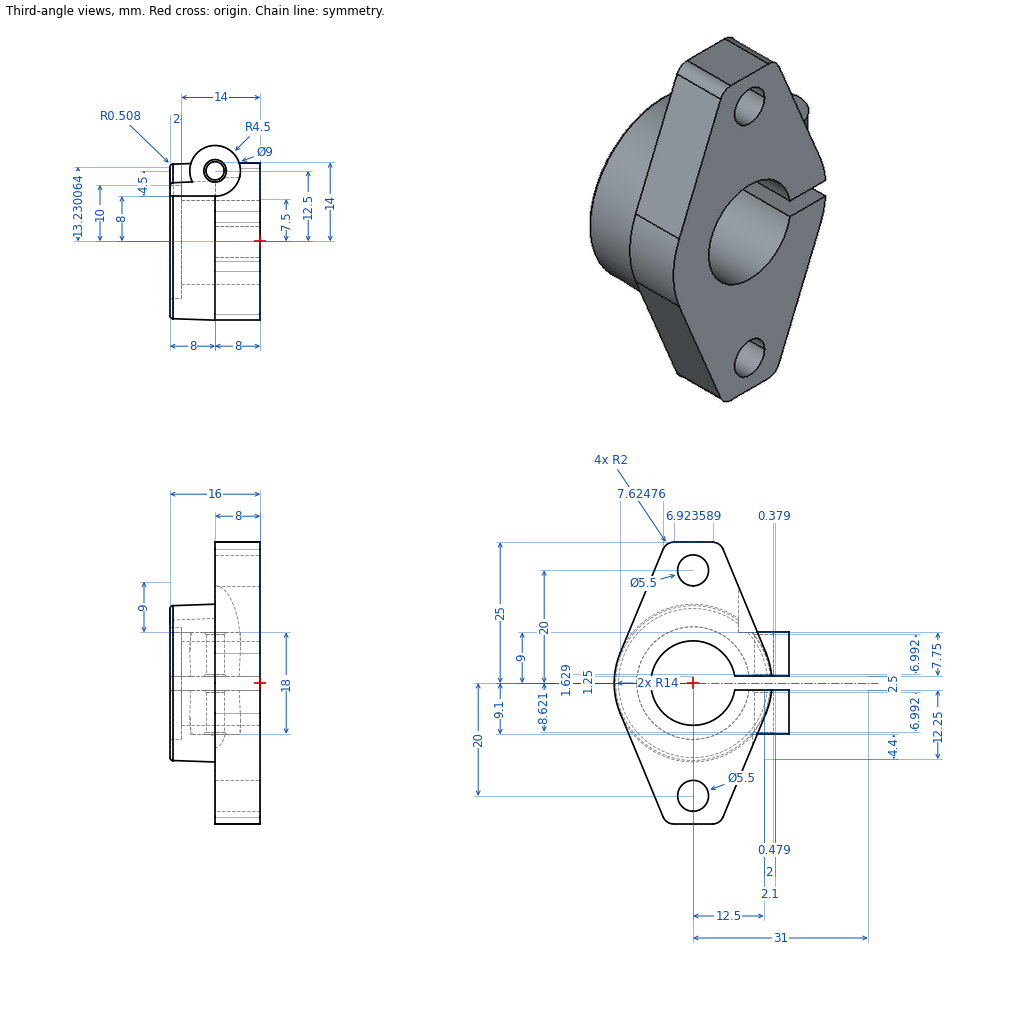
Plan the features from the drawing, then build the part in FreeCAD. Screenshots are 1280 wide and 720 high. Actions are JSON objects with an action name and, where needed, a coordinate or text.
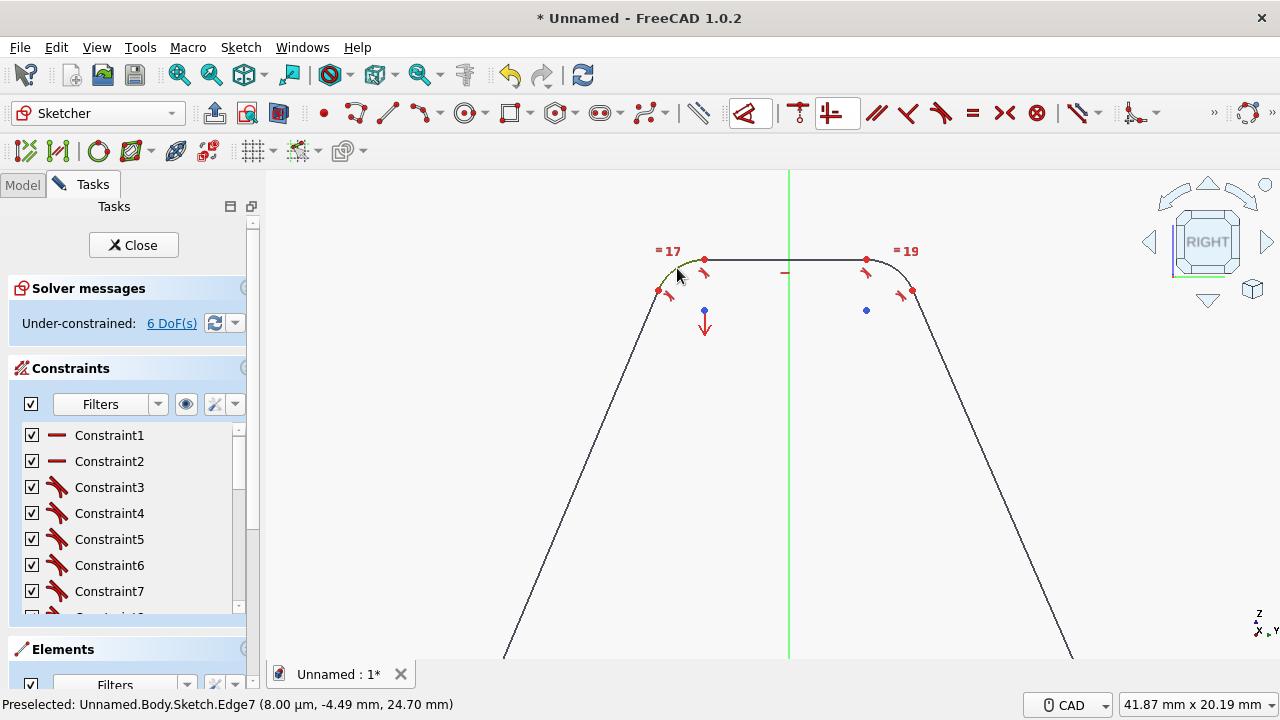
{"action": "key", "text": "k r"}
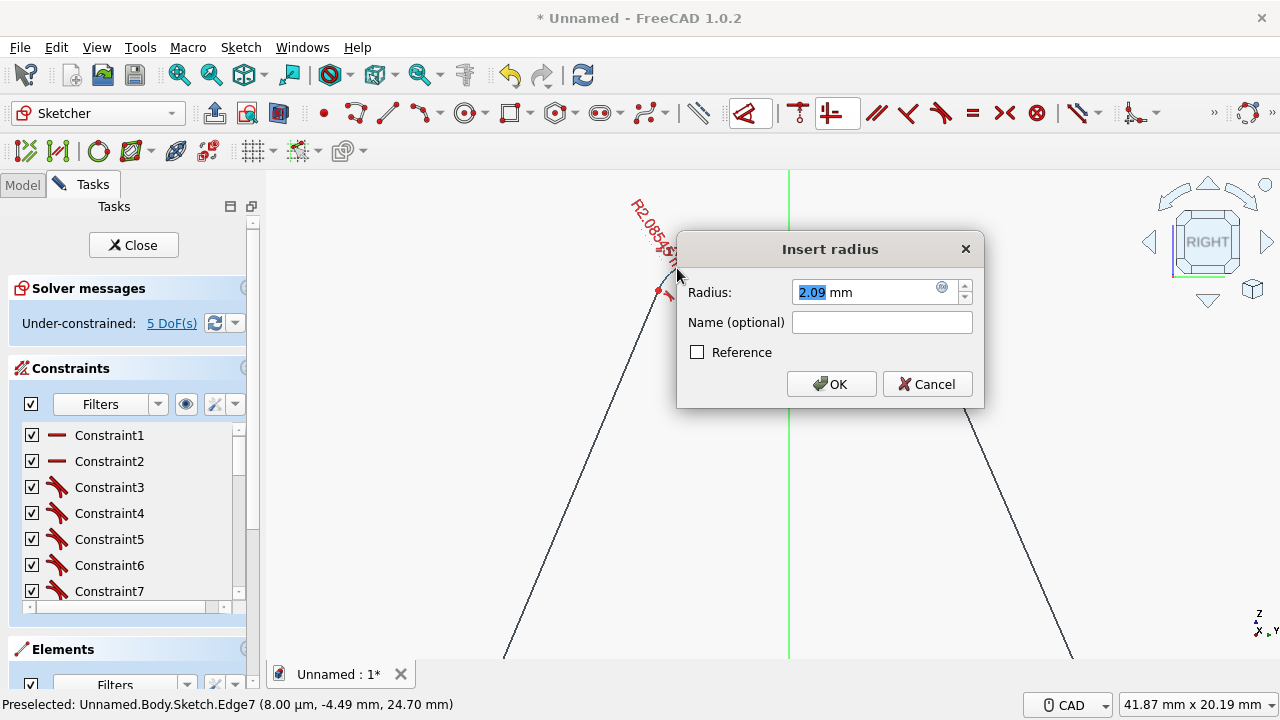
{"action": "type", "text": "2"}
{"action": "key", "text": "Return"}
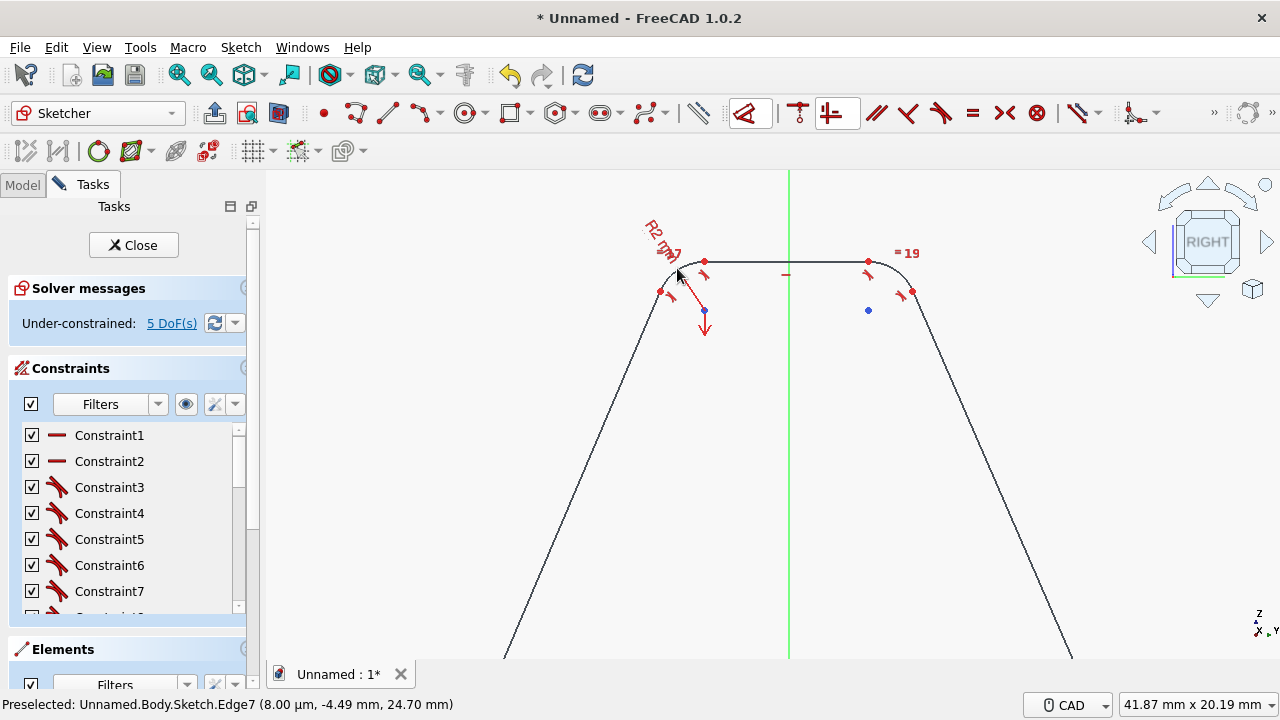
{"action": "scroll", "coordinate": [677, 267], "scroll_direction": "down", "scroll_amount": 7}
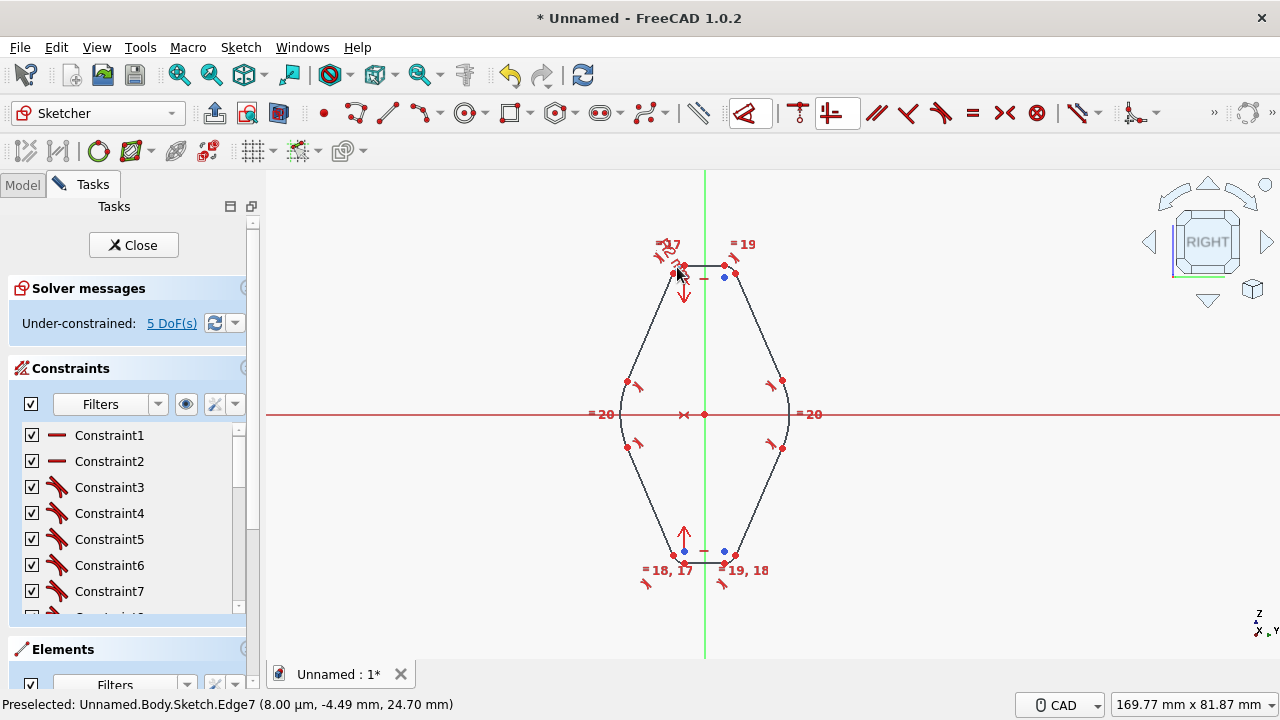
{"action": "left_click", "coordinate": [621, 401]}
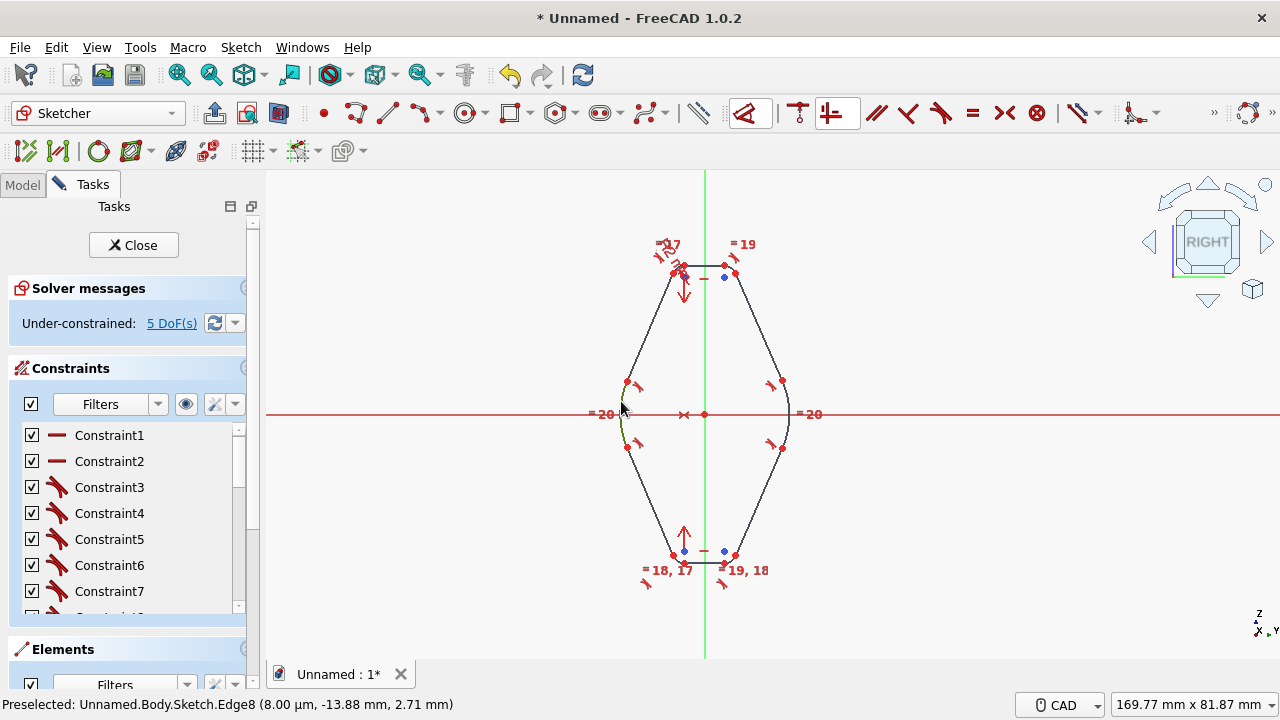
{"action": "key", "text": "k r"}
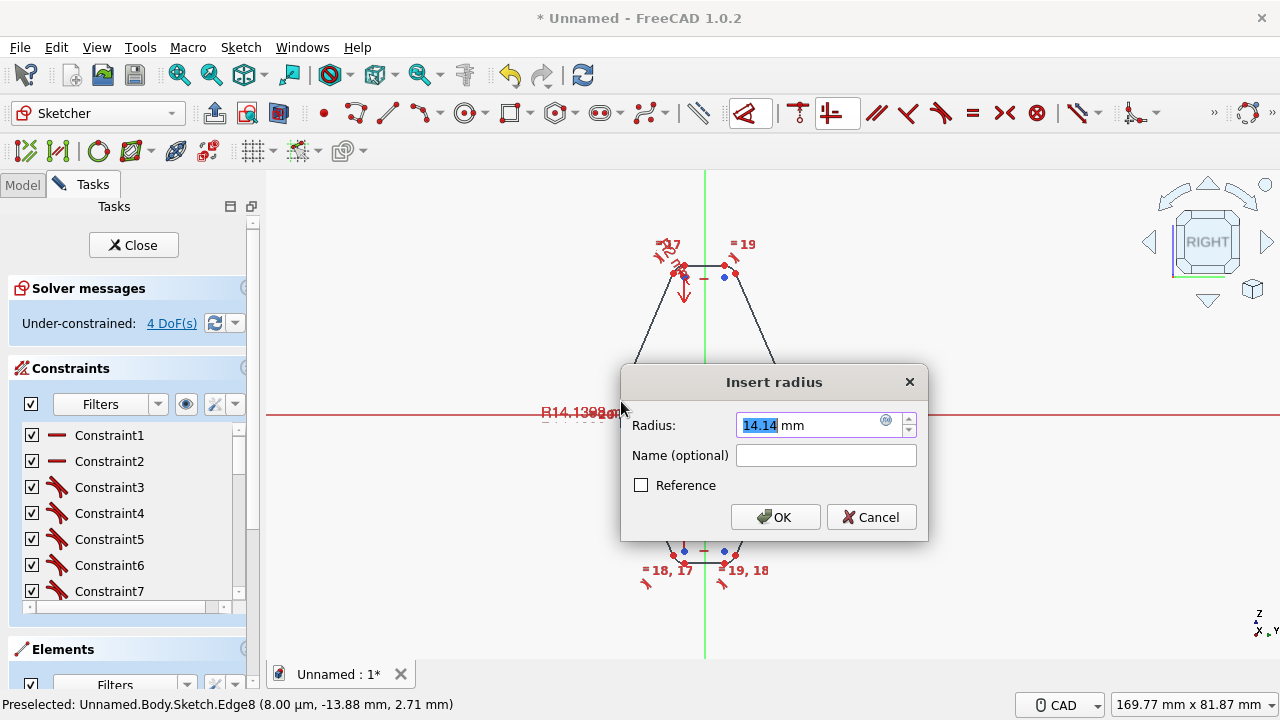
{"action": "type", "text": "14"}
{"action": "key", "text": "Return"}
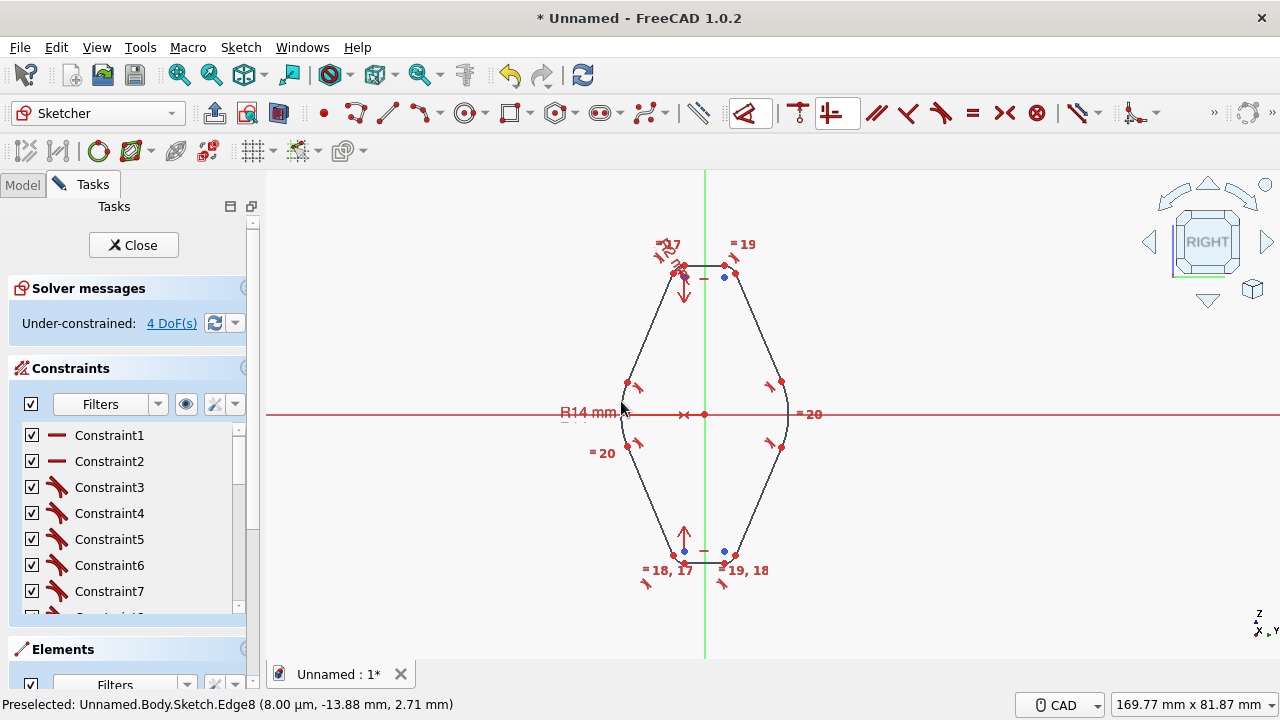
{"action": "left_click", "coordinate": [725, 266]}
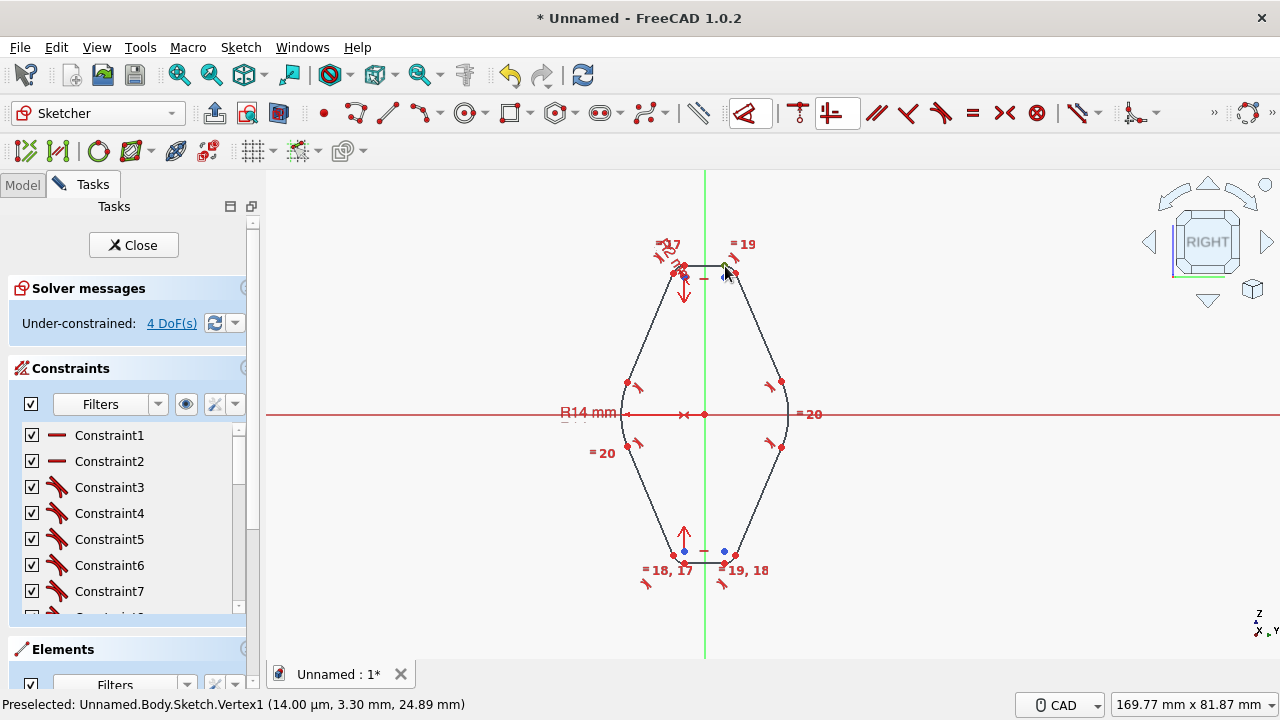
{"action": "left_click", "coordinate": [766, 114]}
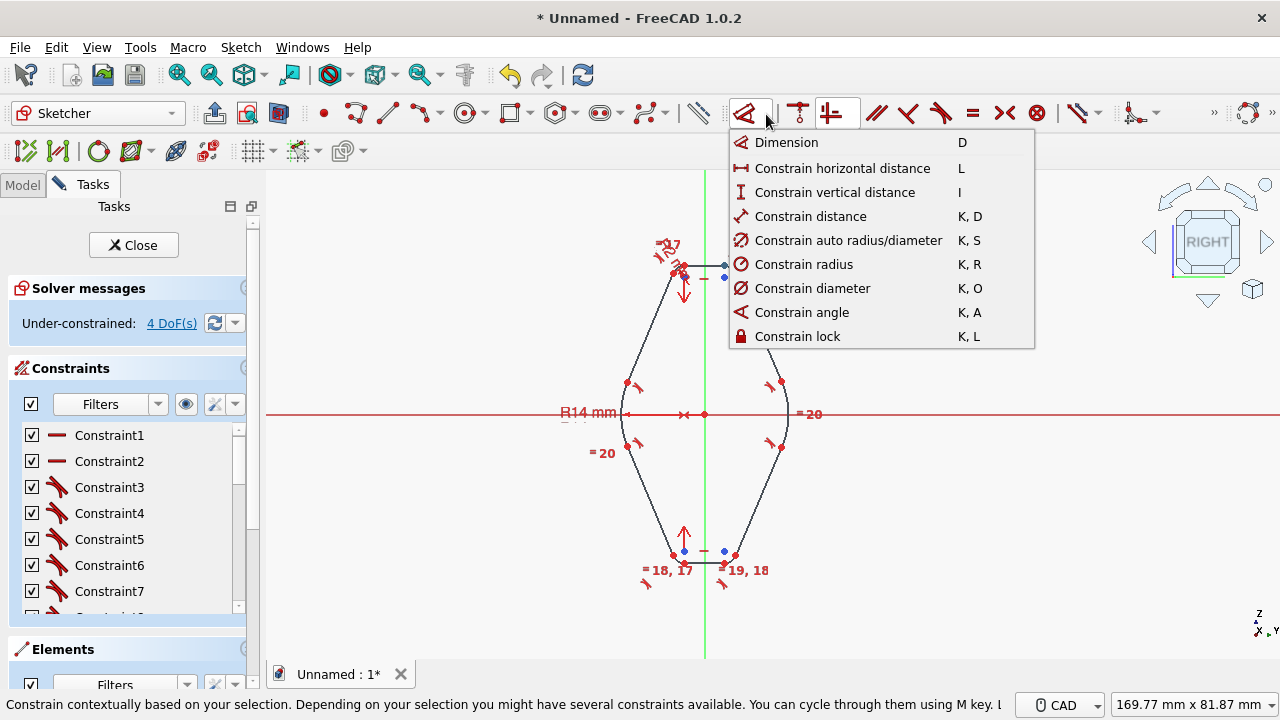
{"action": "left_click", "coordinate": [882, 192]}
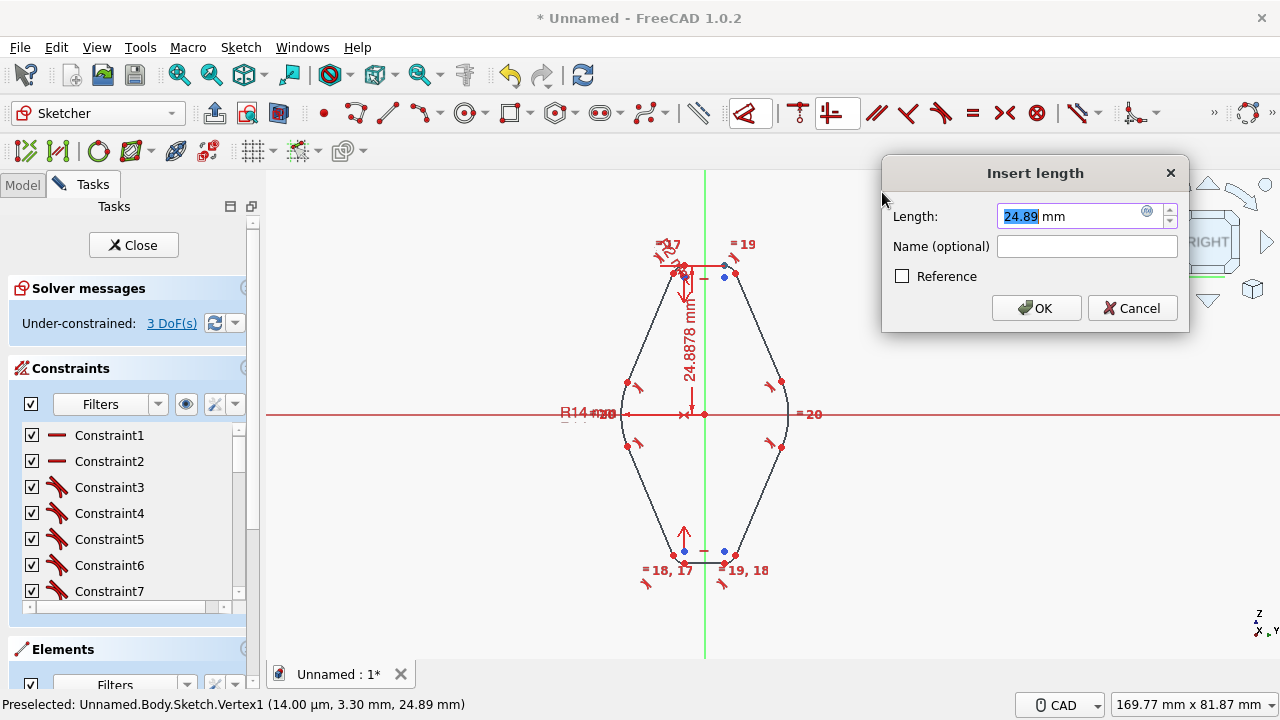
{"action": "type", "text": "25"}
{"action": "key", "text": "Return"}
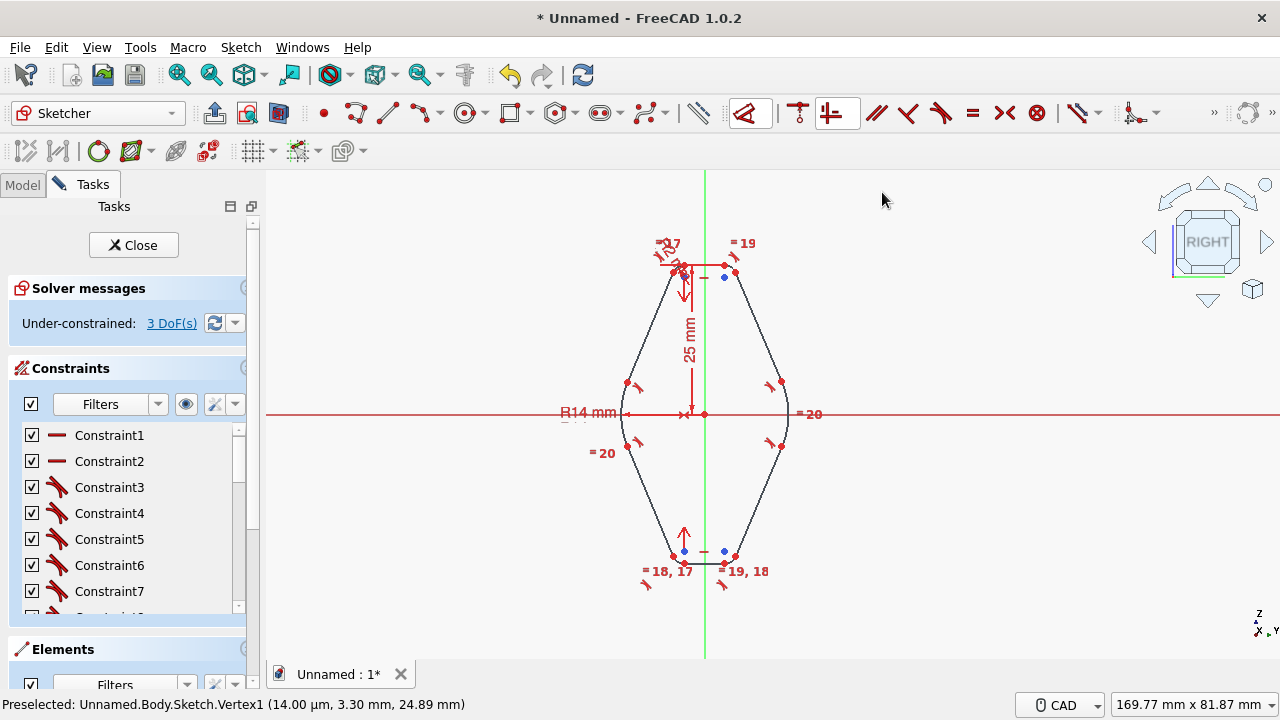
{"action": "left_click", "coordinate": [708, 265]}